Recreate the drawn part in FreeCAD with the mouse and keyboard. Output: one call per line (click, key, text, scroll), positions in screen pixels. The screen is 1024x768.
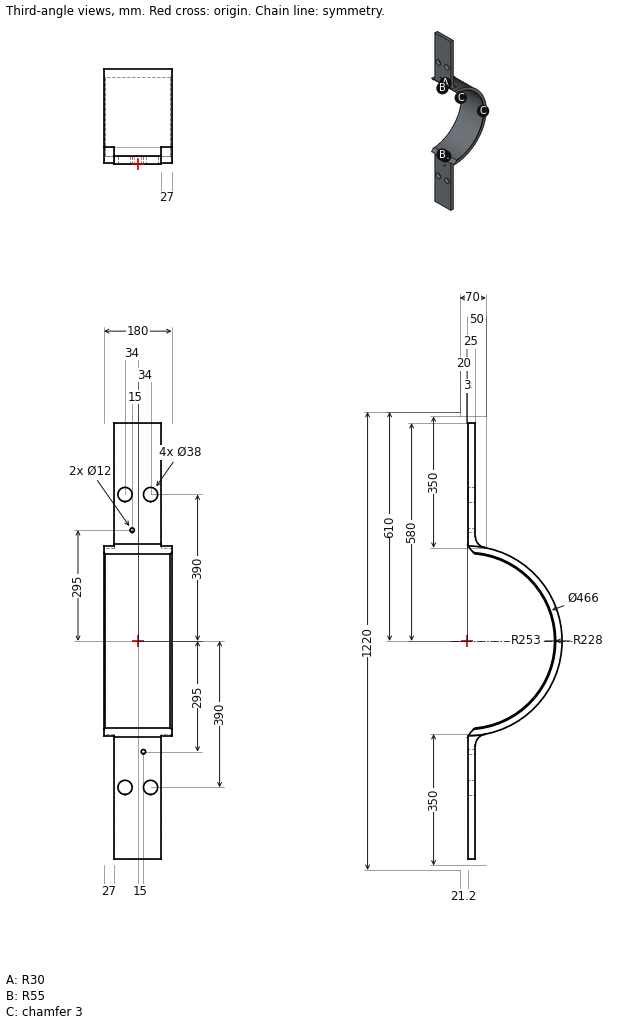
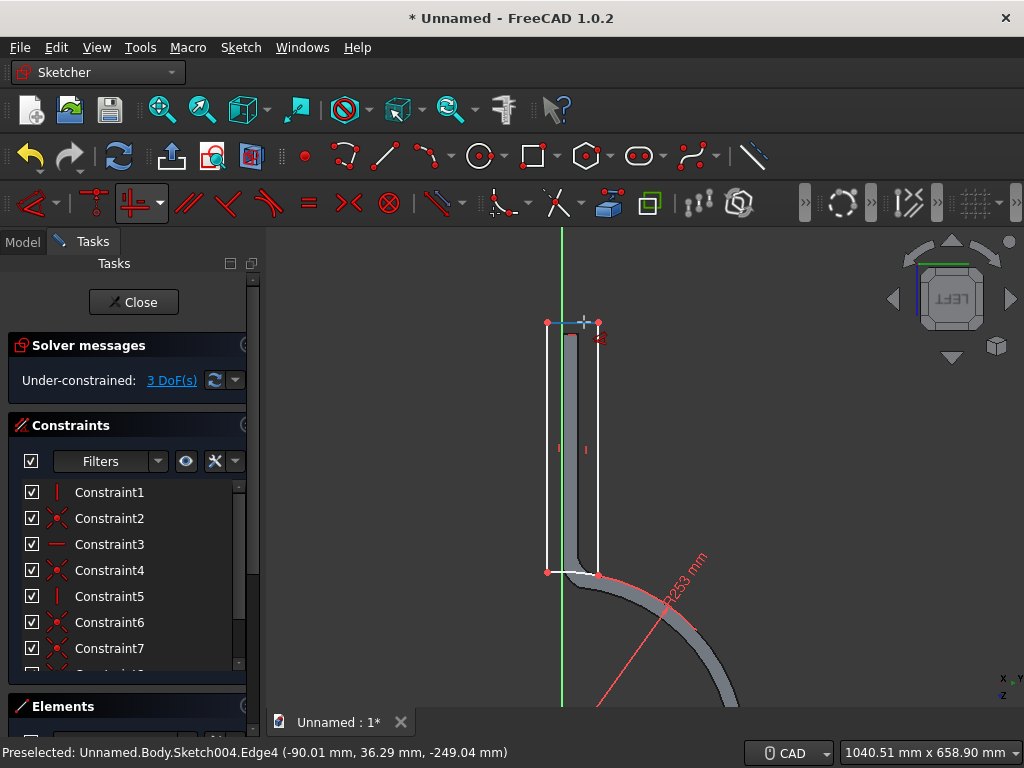
click(583, 323)
click(585, 289)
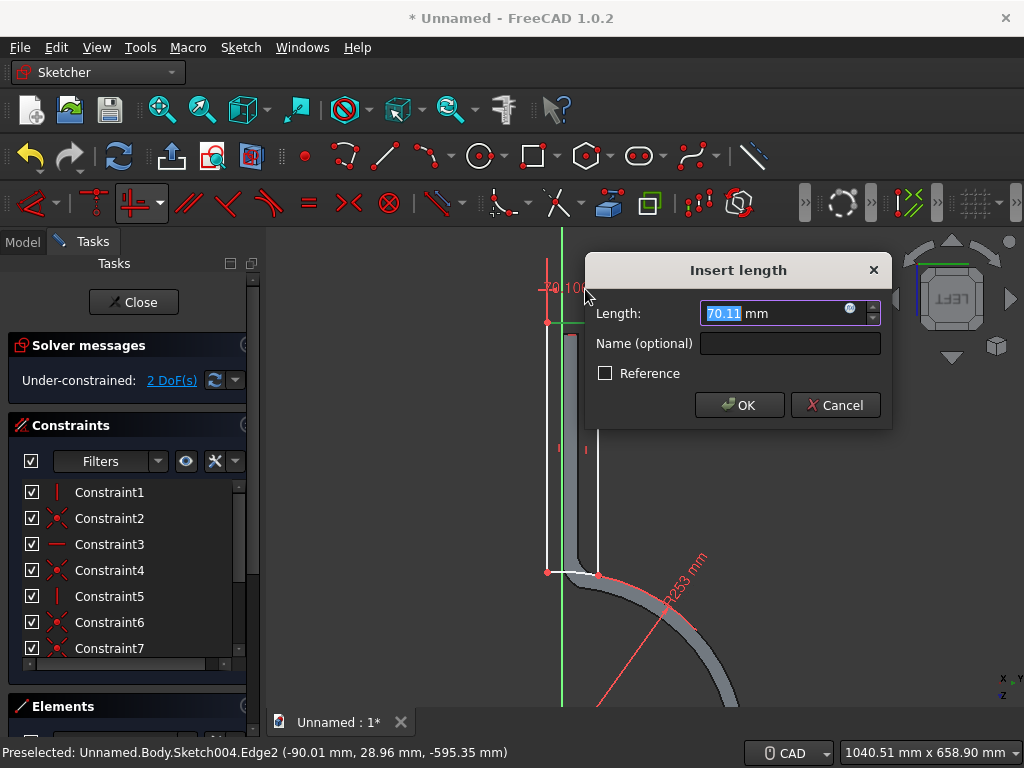
text(70)
key(Return)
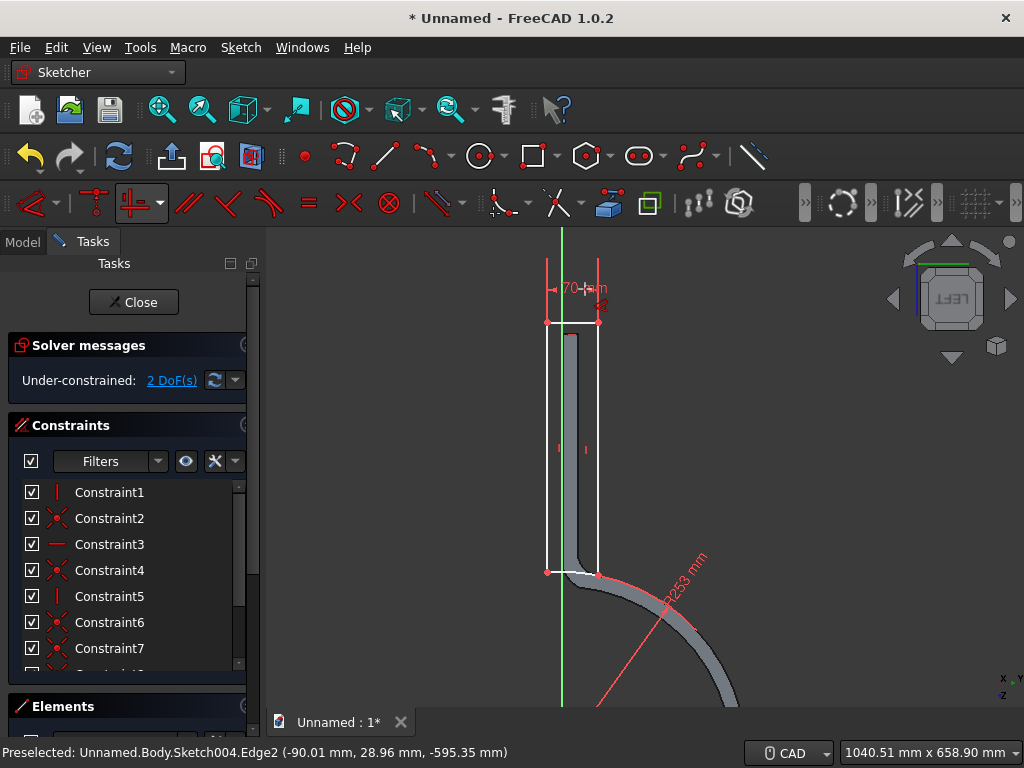
click(598, 500)
click(632, 449)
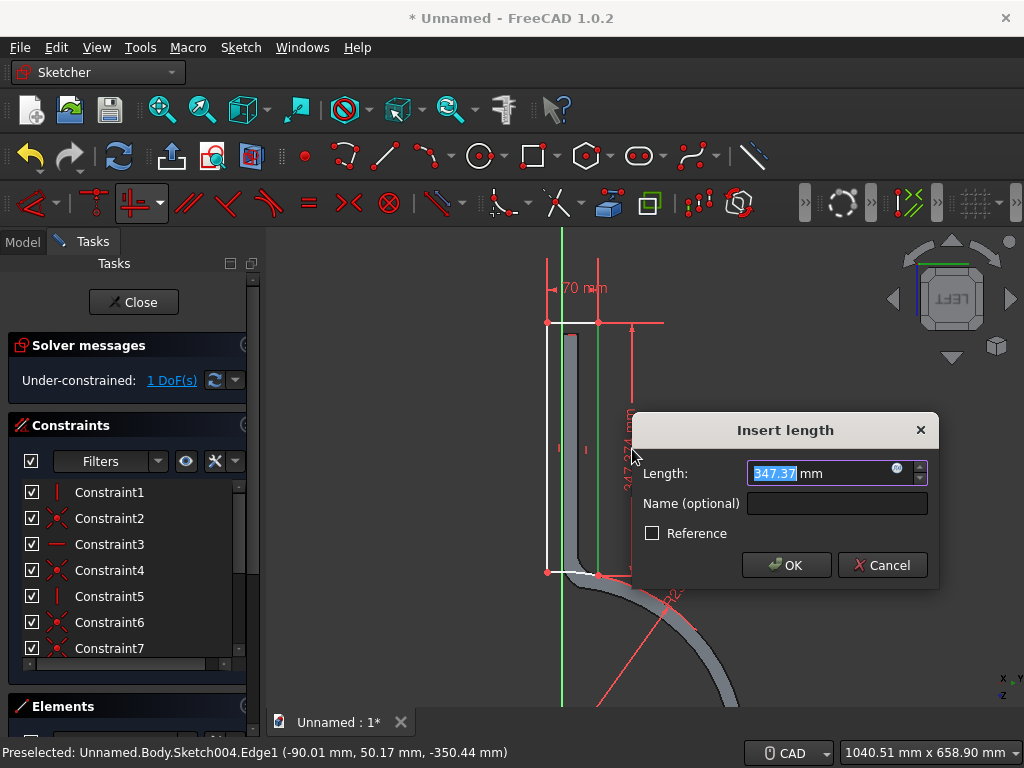
text(350)
key(Return)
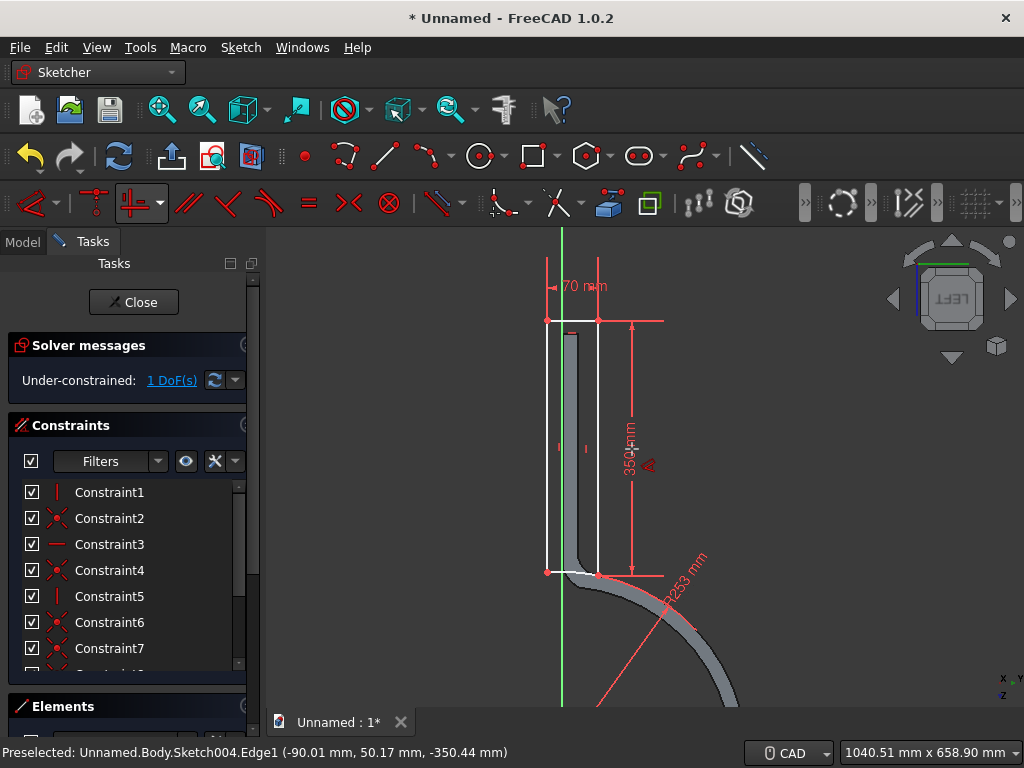
click(598, 576)
click(580, 542)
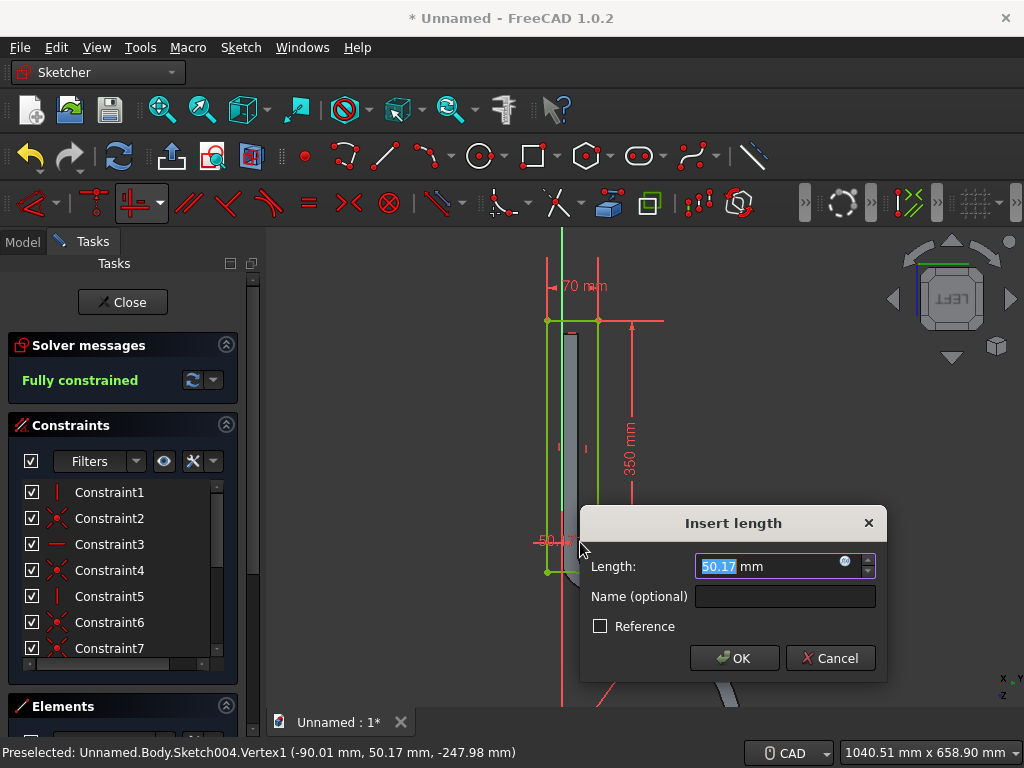
text(50)
key(Return)
key(Escape)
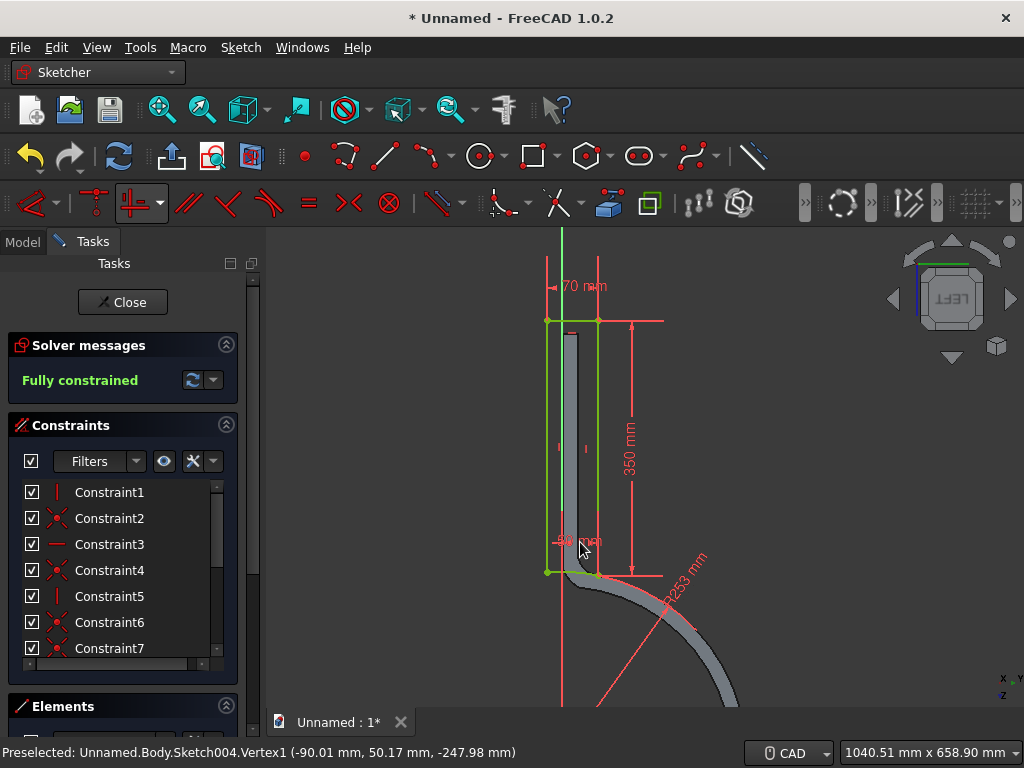
click(123, 302)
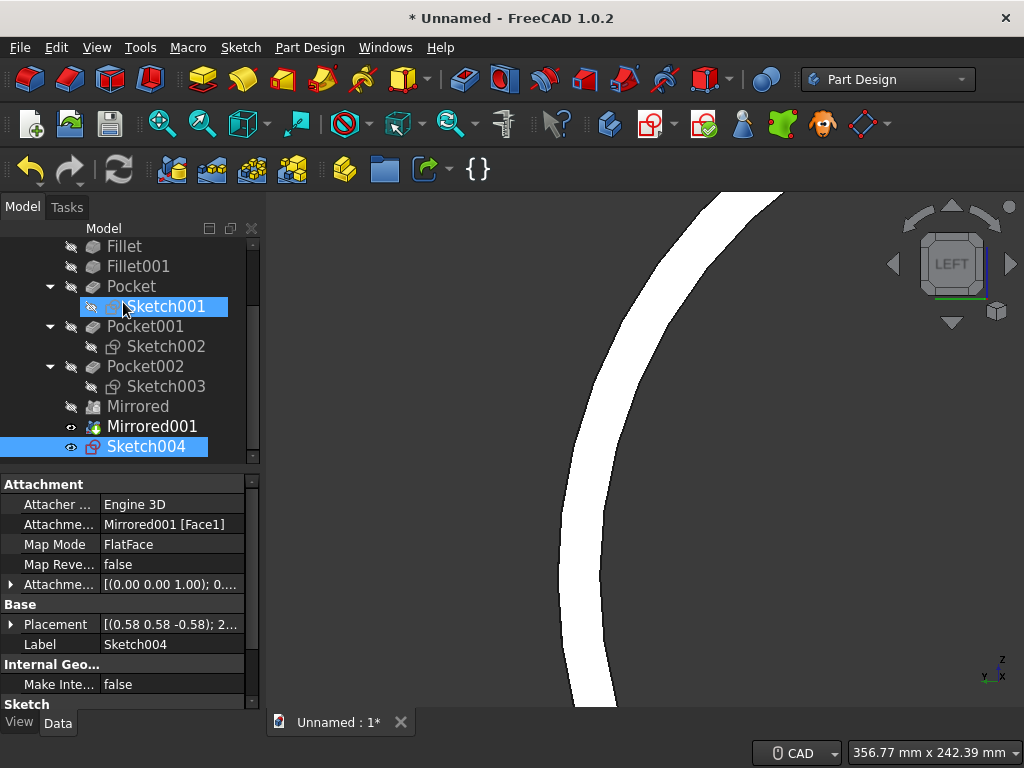
click(466, 80)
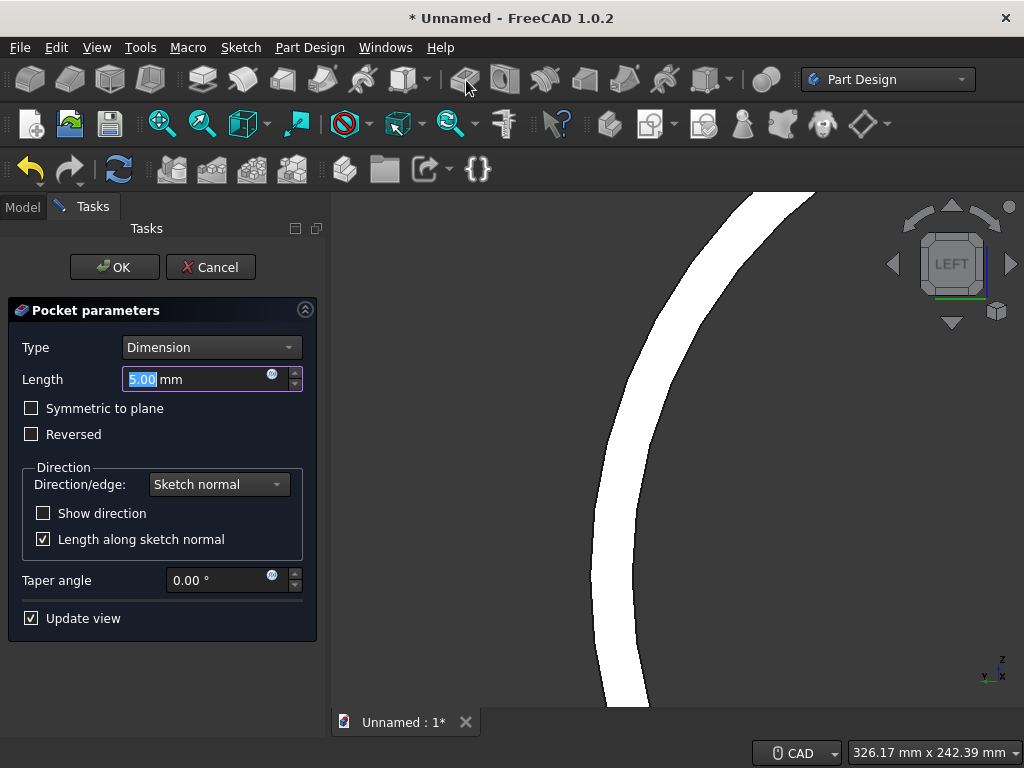
text(27)
key(Tab)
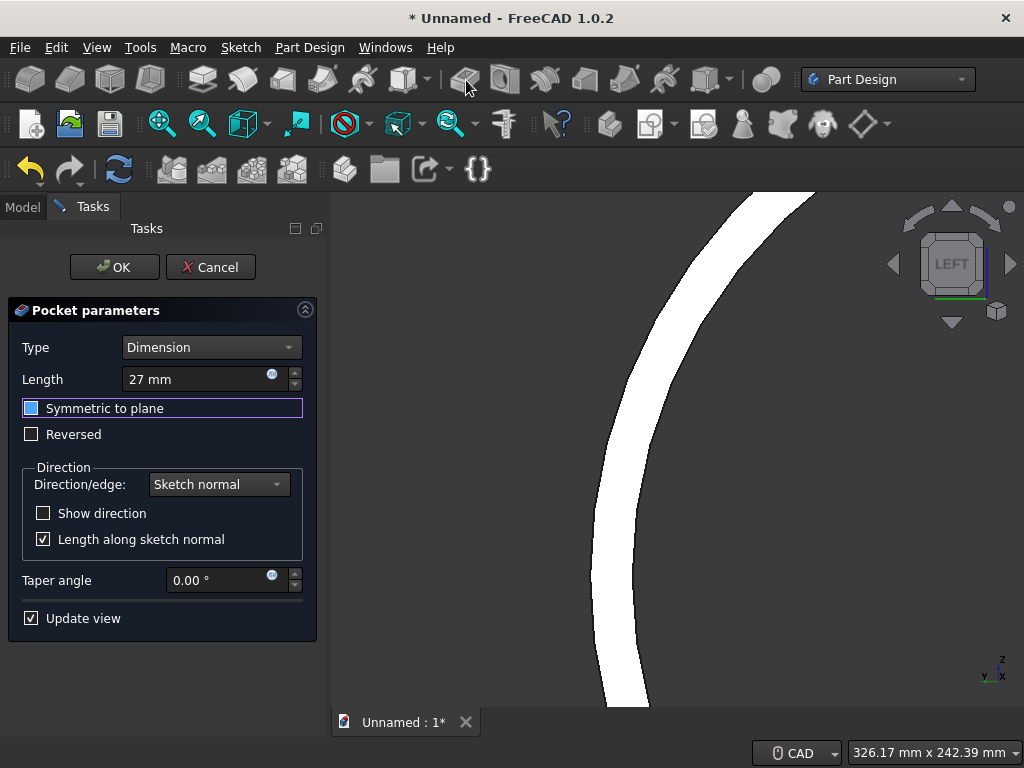
click(115, 267)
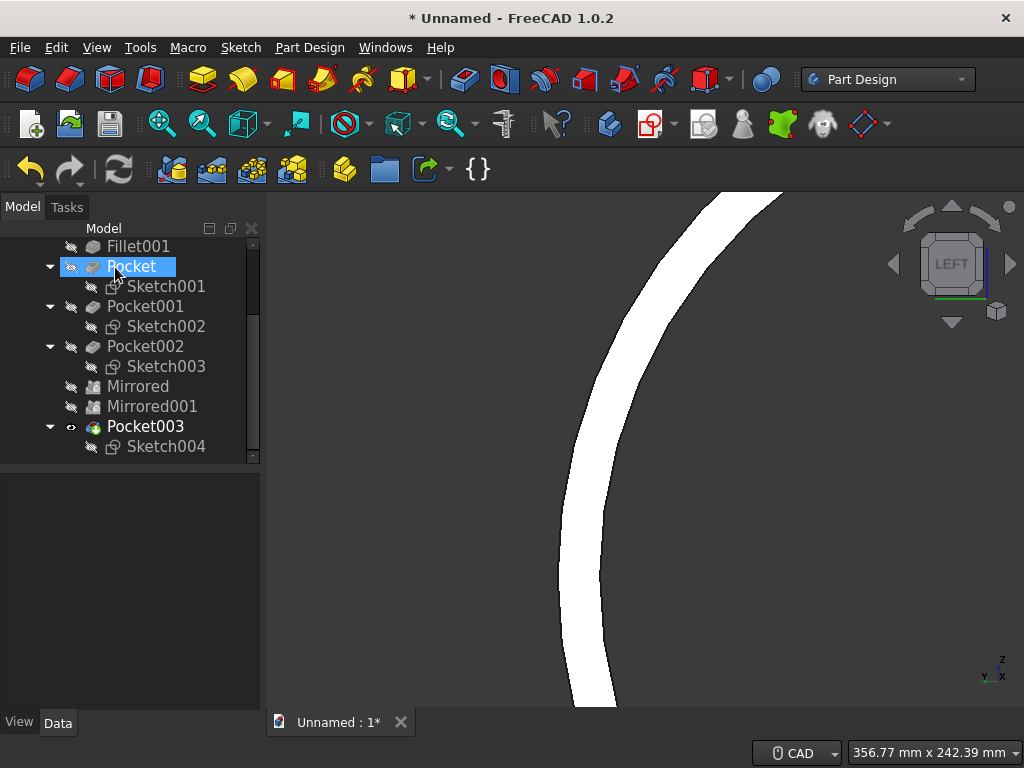
click(164, 124)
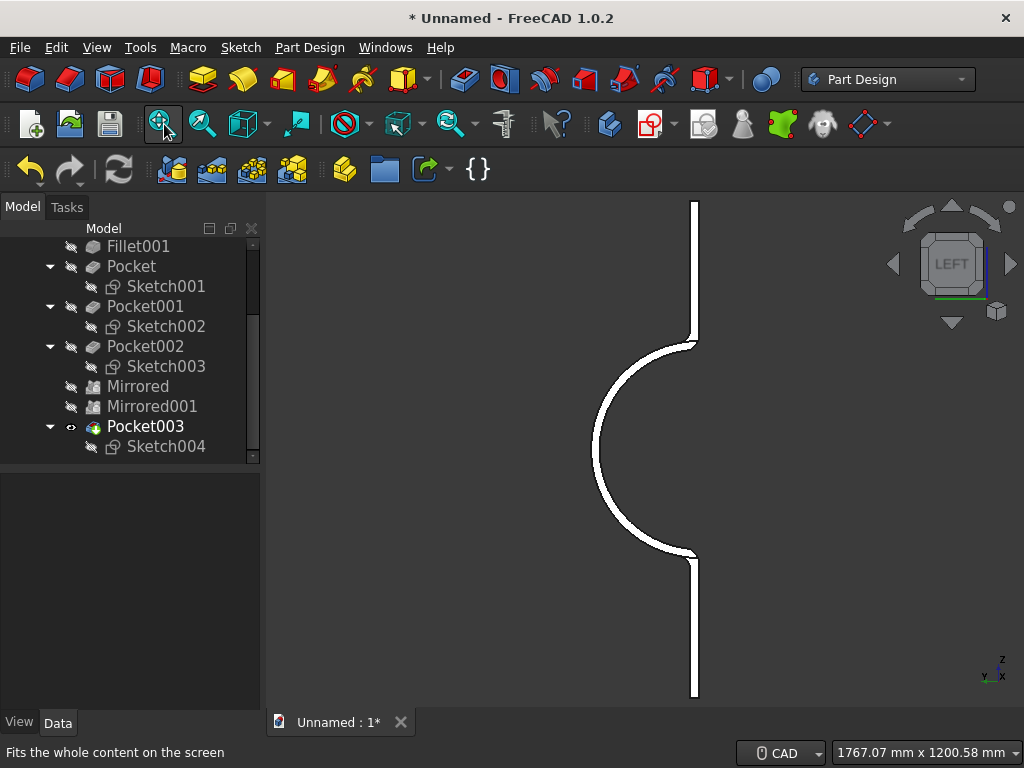
click(650, 124)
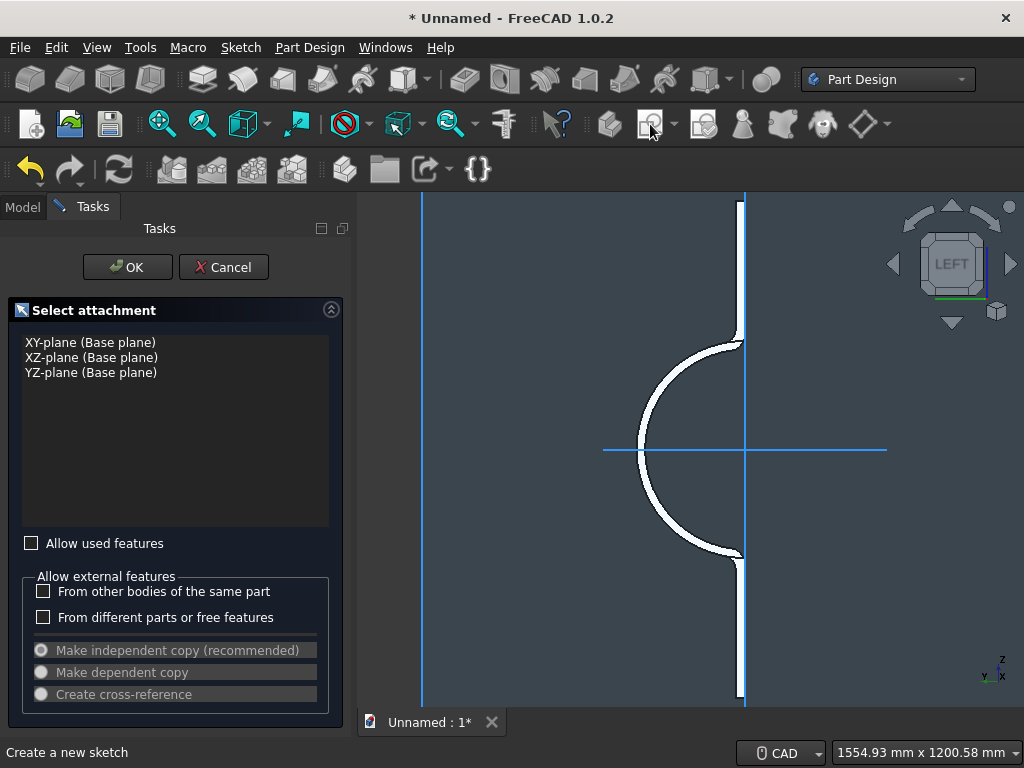
click(82, 358)